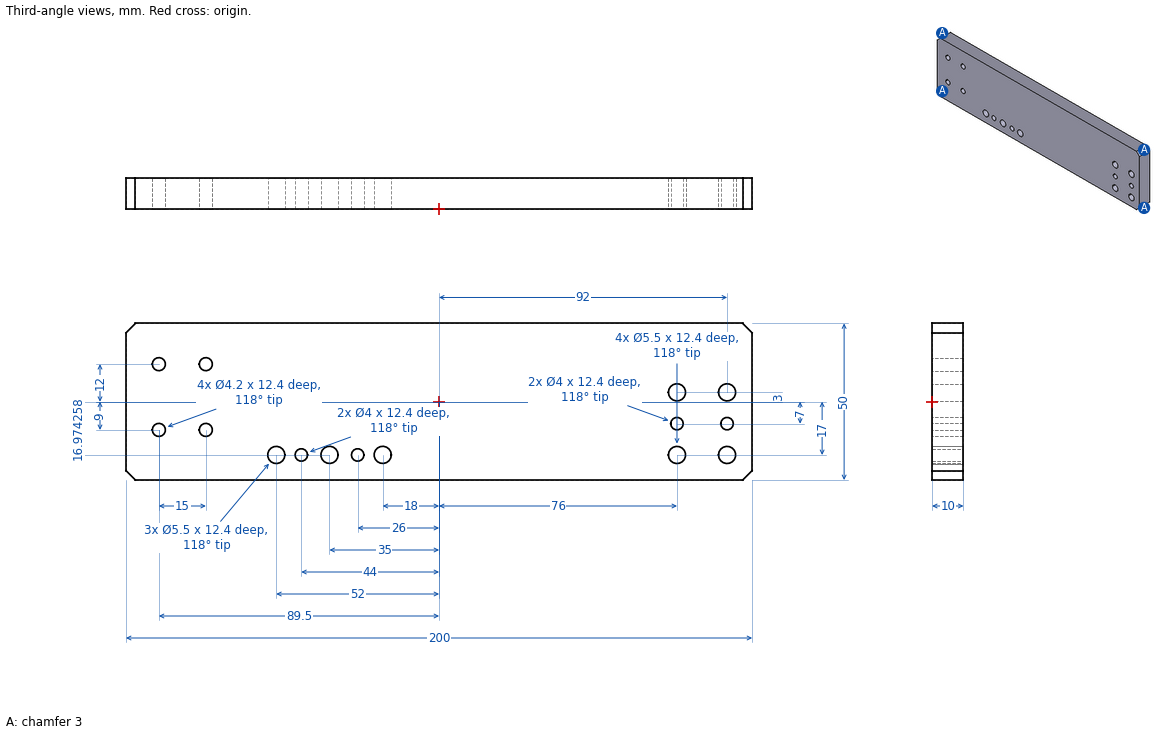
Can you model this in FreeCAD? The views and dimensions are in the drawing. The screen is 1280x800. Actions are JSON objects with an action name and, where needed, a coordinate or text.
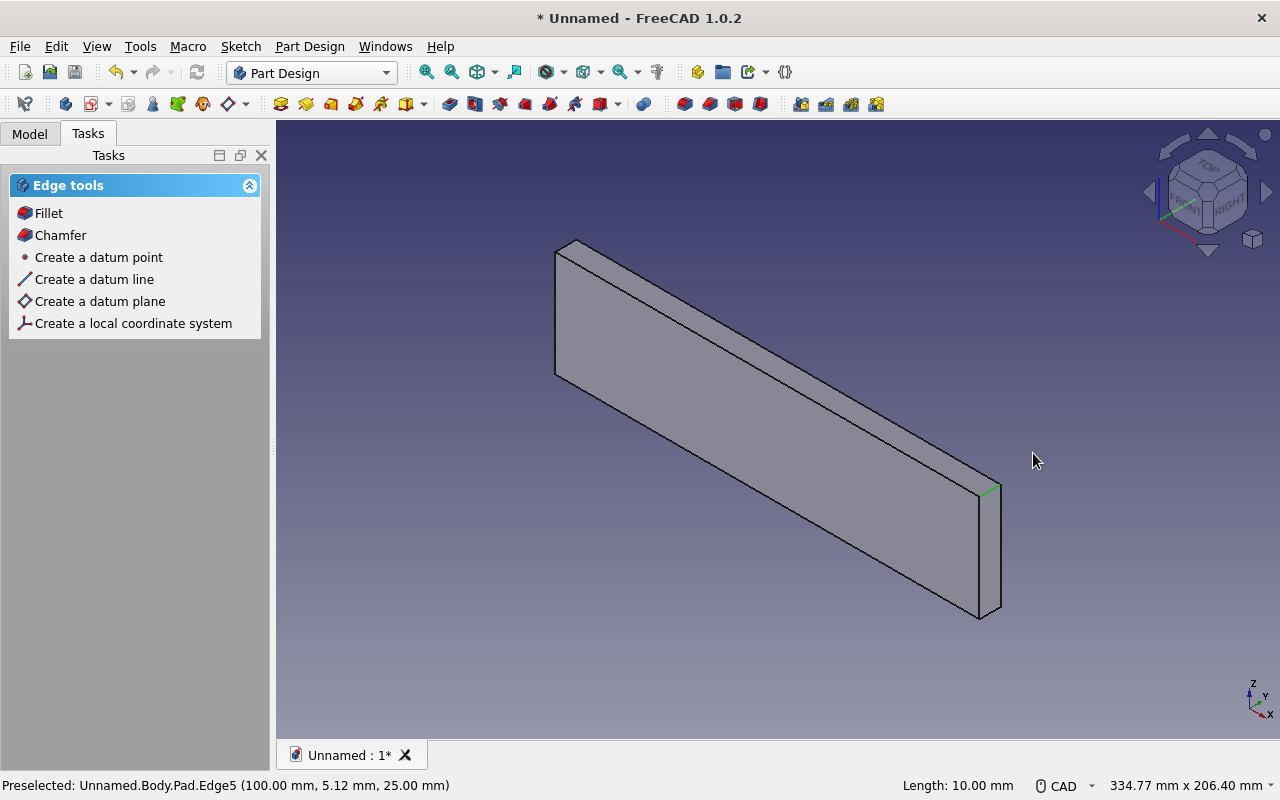
{"action": "key", "text": "2"}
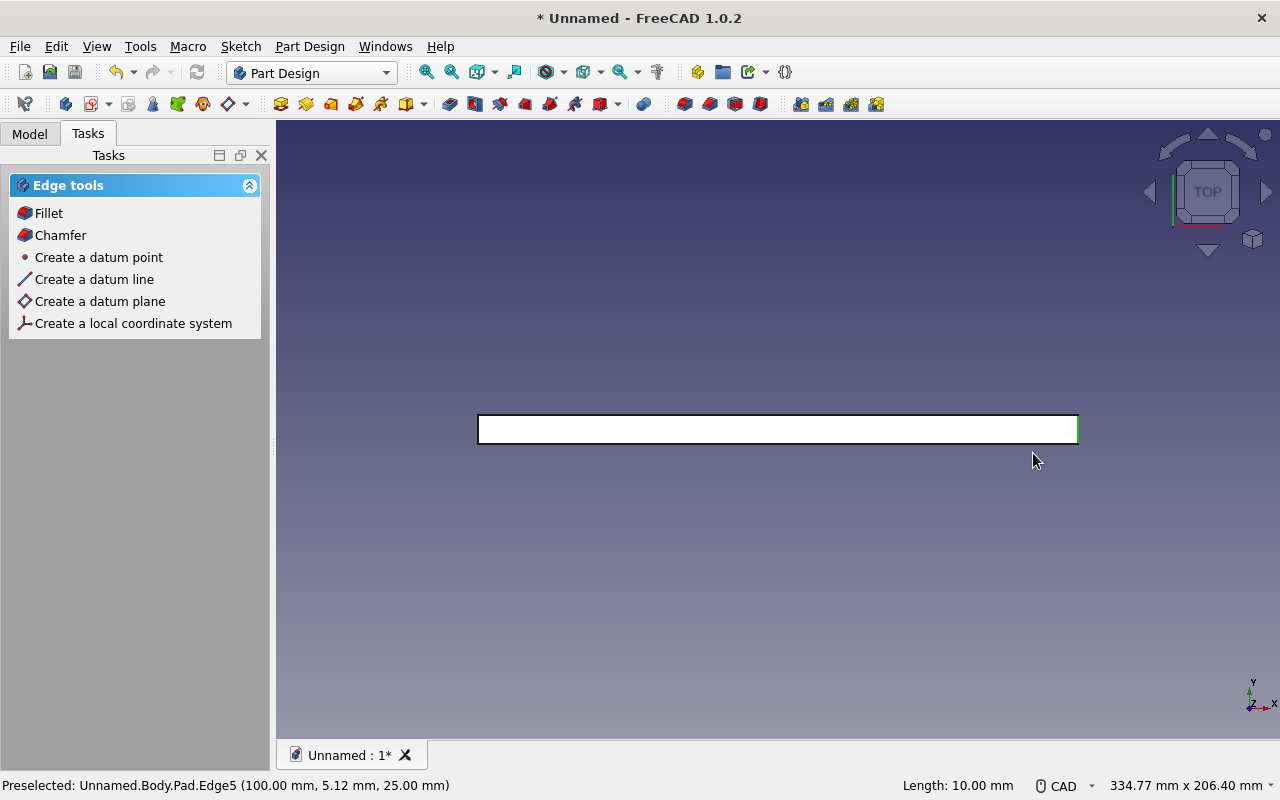
{"action": "left_click", "coordinate": [478, 429], "text": "ctrl"}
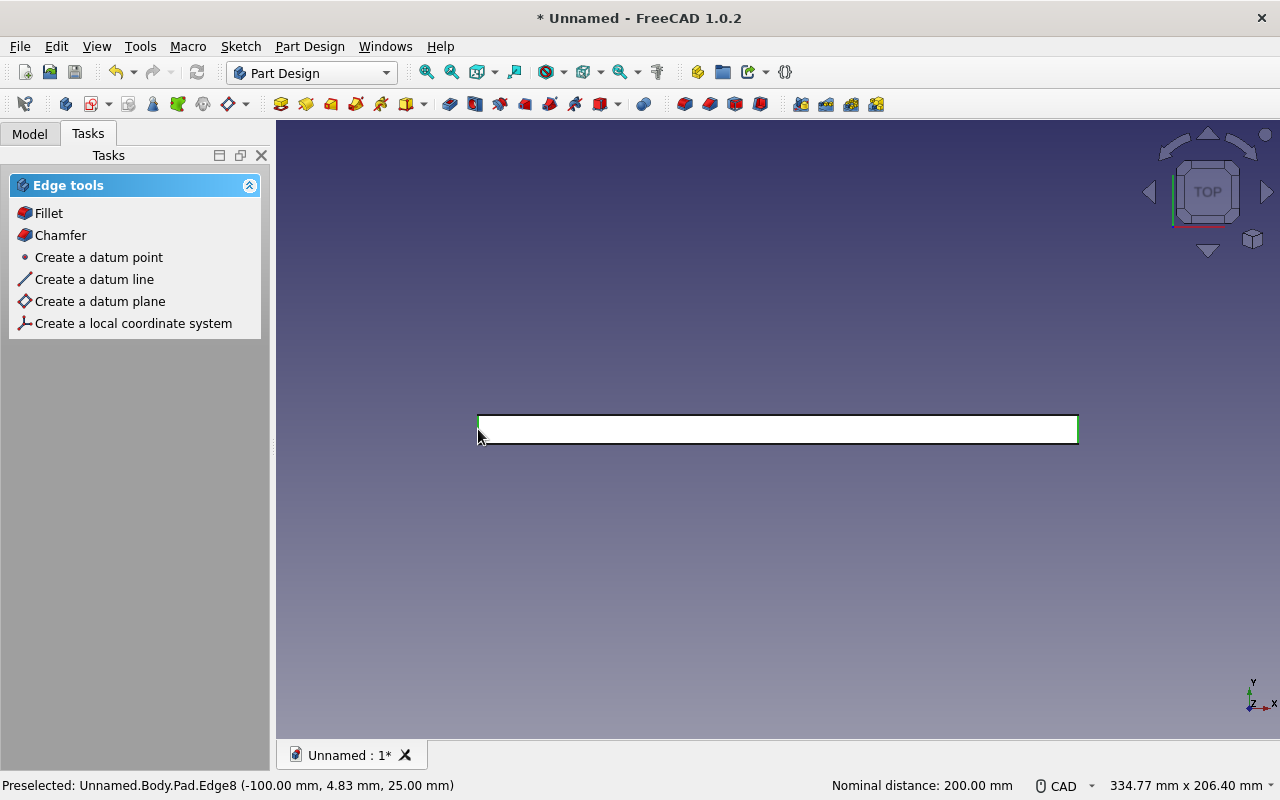
{"action": "key", "text": "1"}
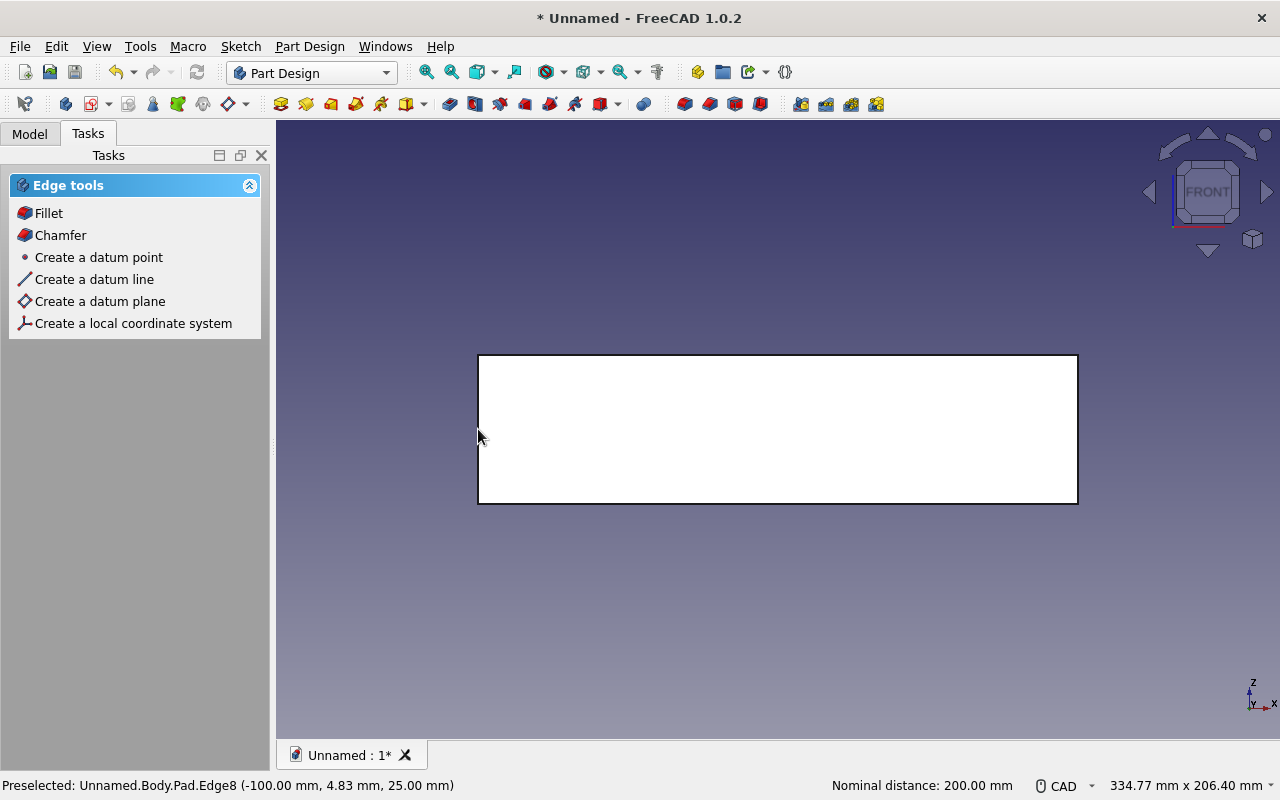
{"action": "key", "text": "3"}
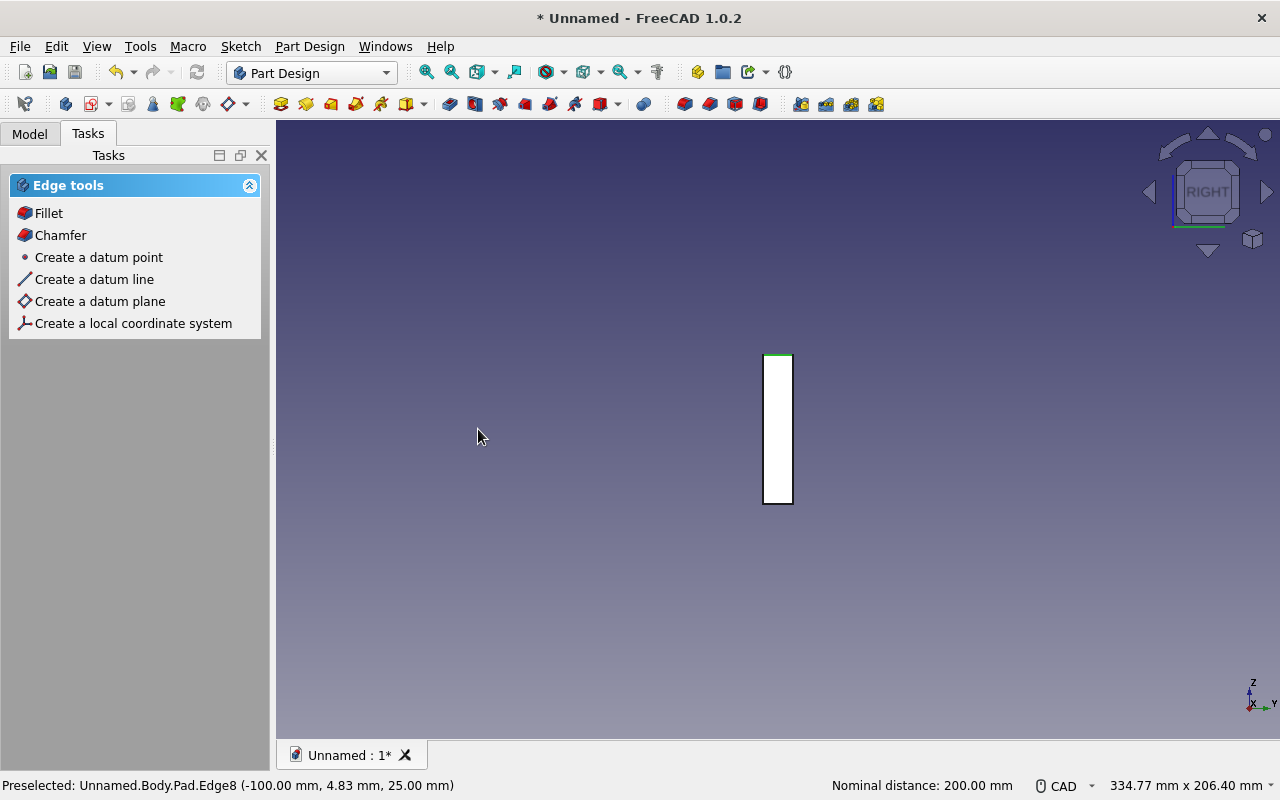
{"action": "left_click", "coordinate": [427, 72]}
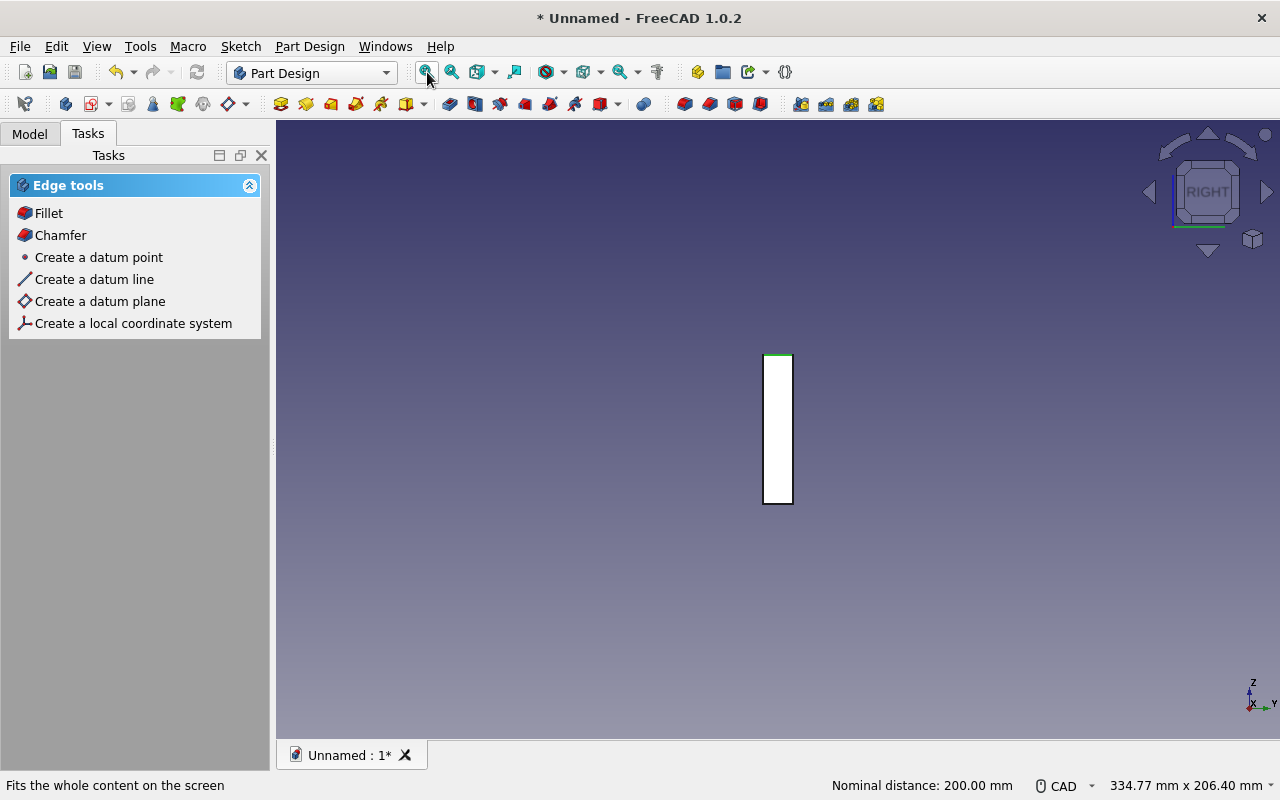
{"action": "left_click", "coordinate": [778, 503], "text": "ctrl"}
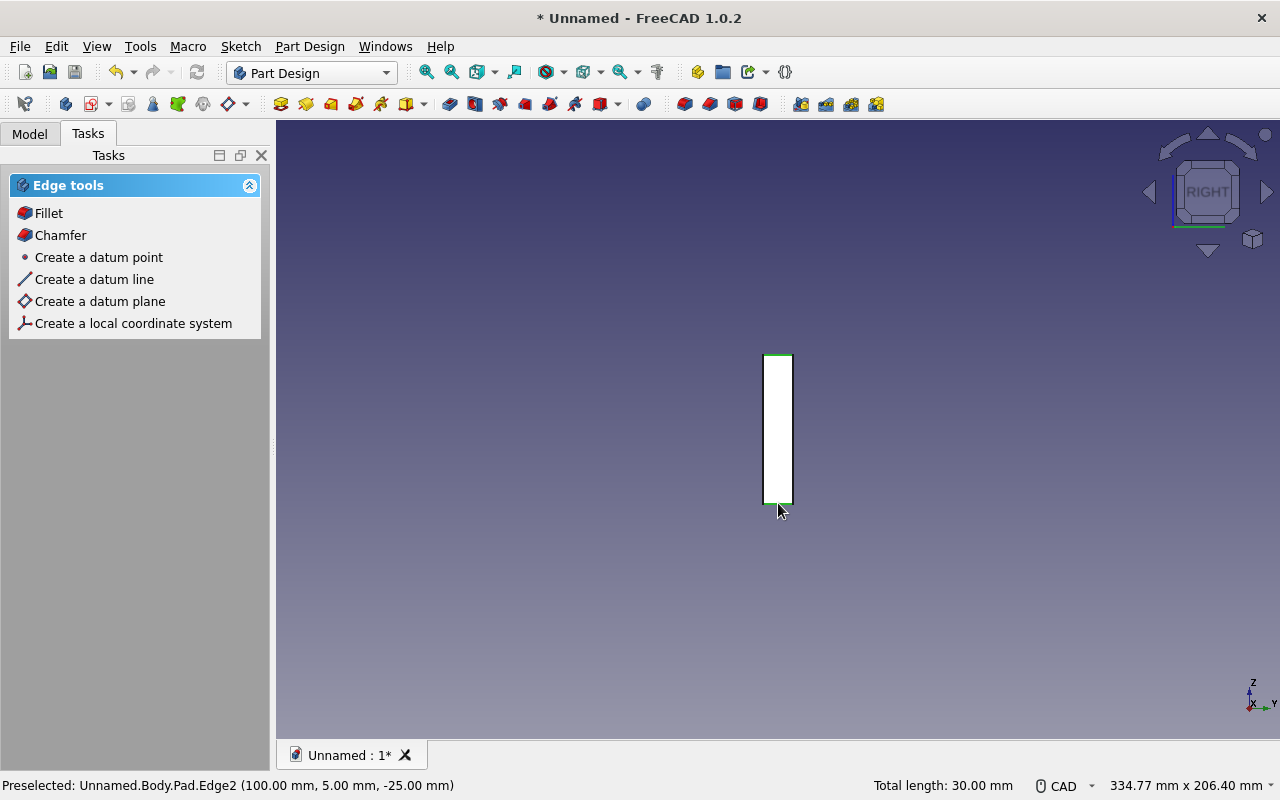
{"action": "key", "text": "5"}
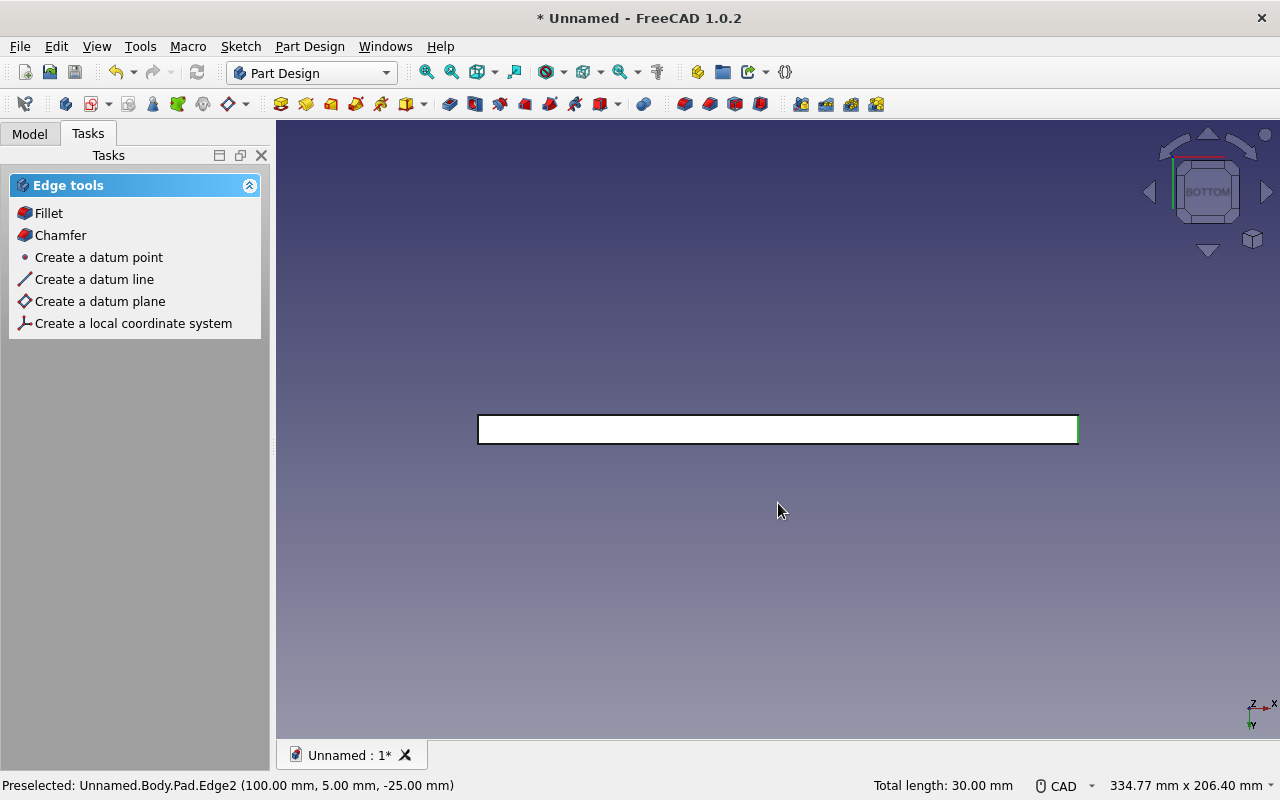
{"action": "left_click", "coordinate": [478, 428], "text": "ctrl"}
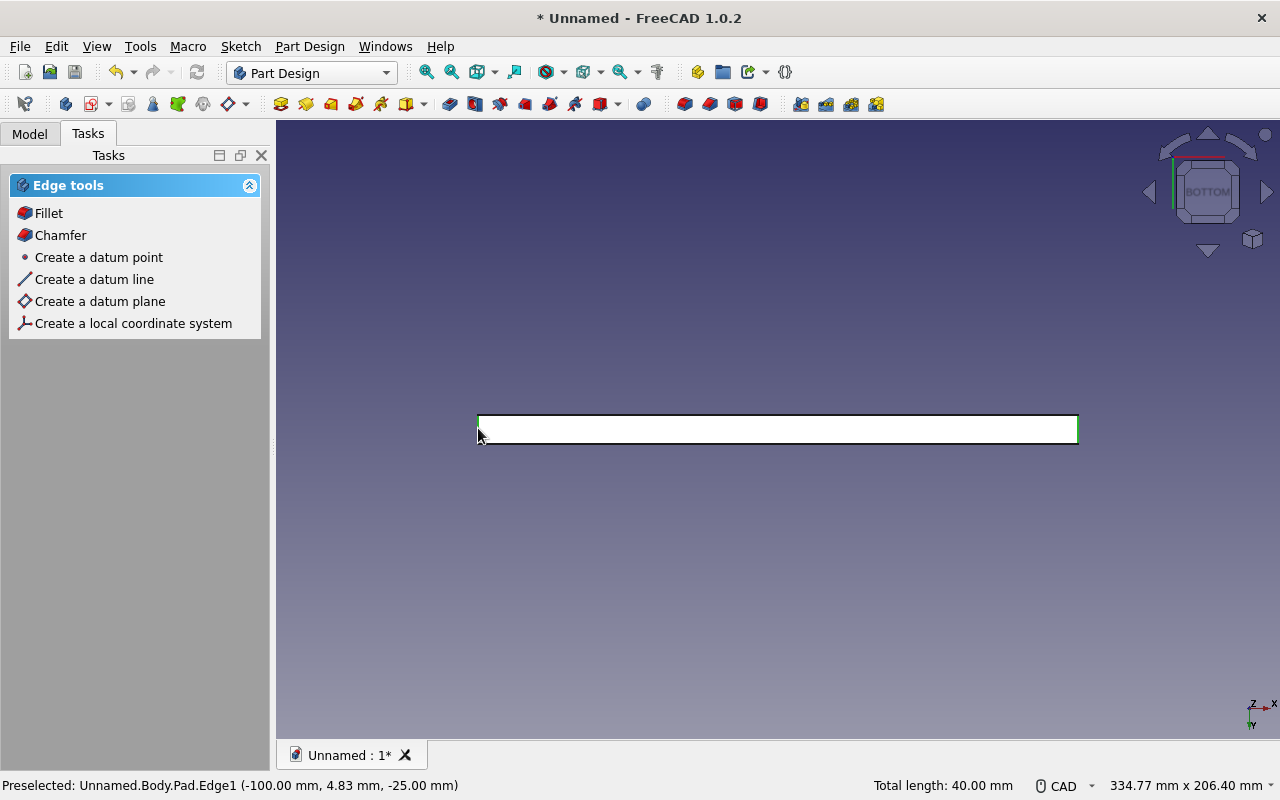
{"action": "left_click", "coordinate": [710, 104]}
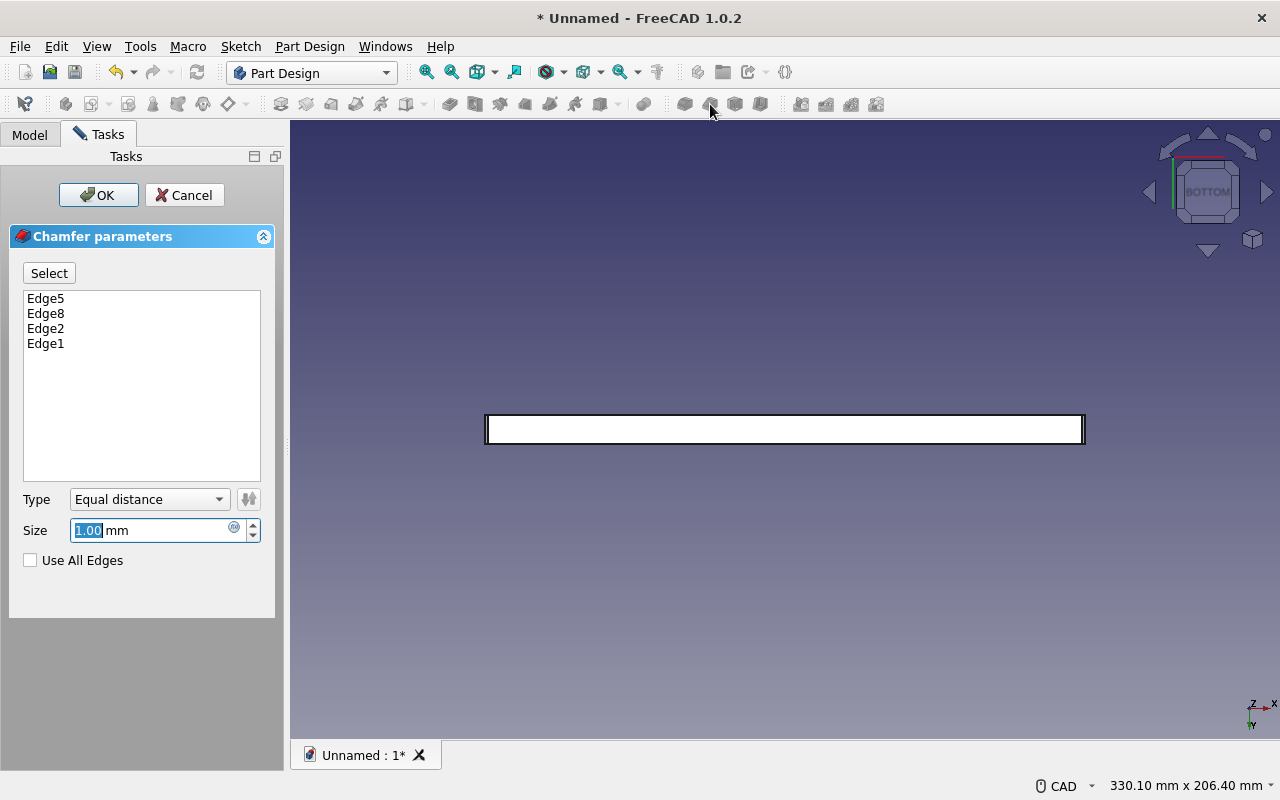
{"action": "type", "text": "3"}
{"action": "key", "text": "Tab"}